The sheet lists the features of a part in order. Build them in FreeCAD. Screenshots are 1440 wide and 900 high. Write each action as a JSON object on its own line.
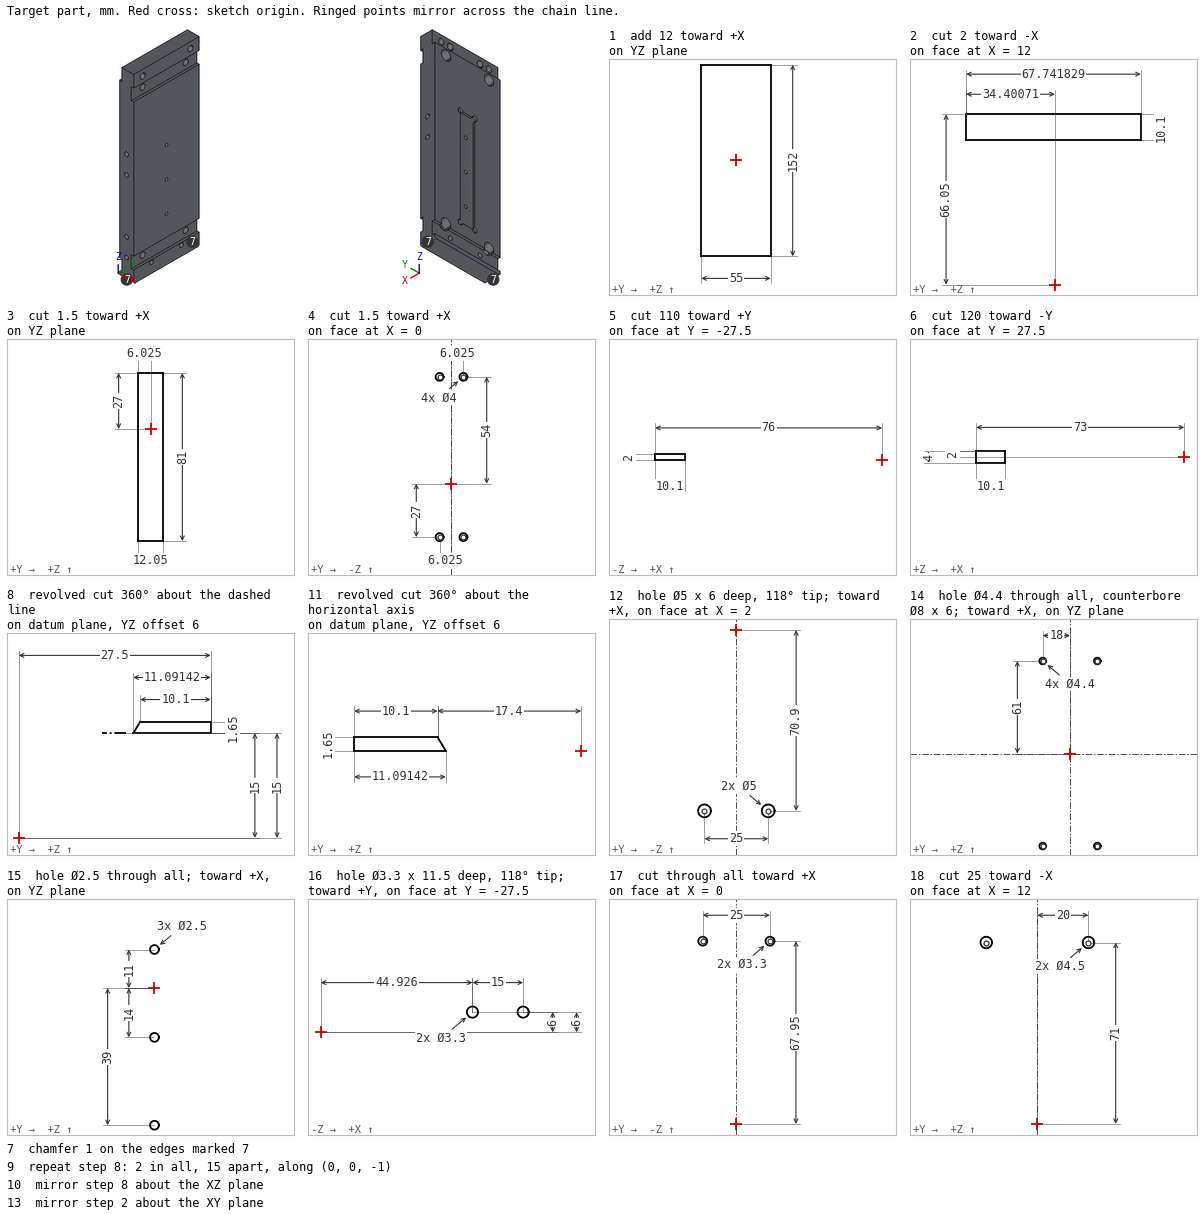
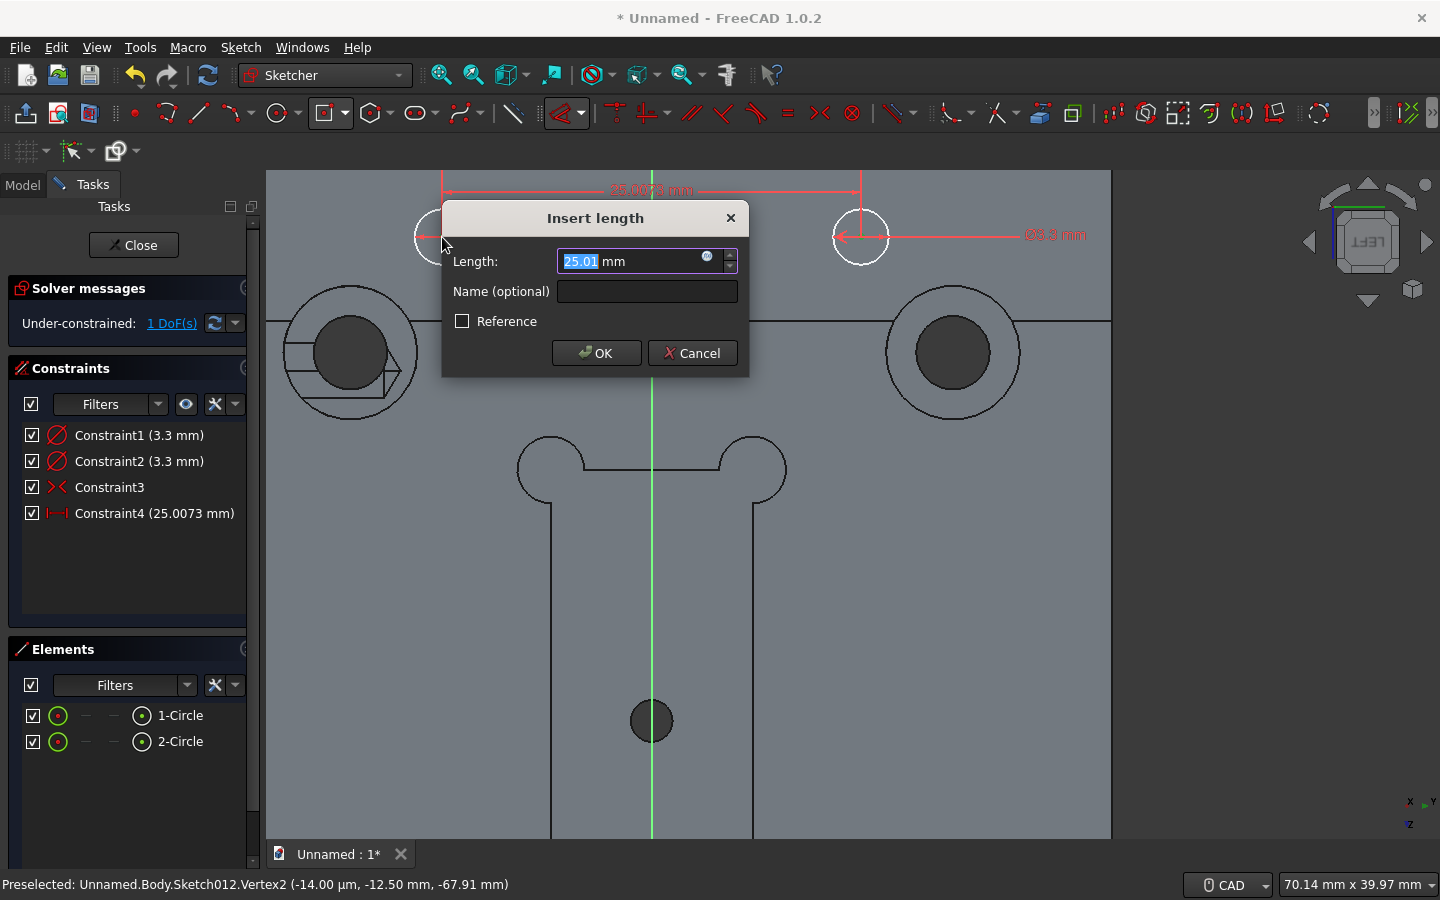
{"action": "type", "text": "25"}
{"action": "key", "text": "Return"}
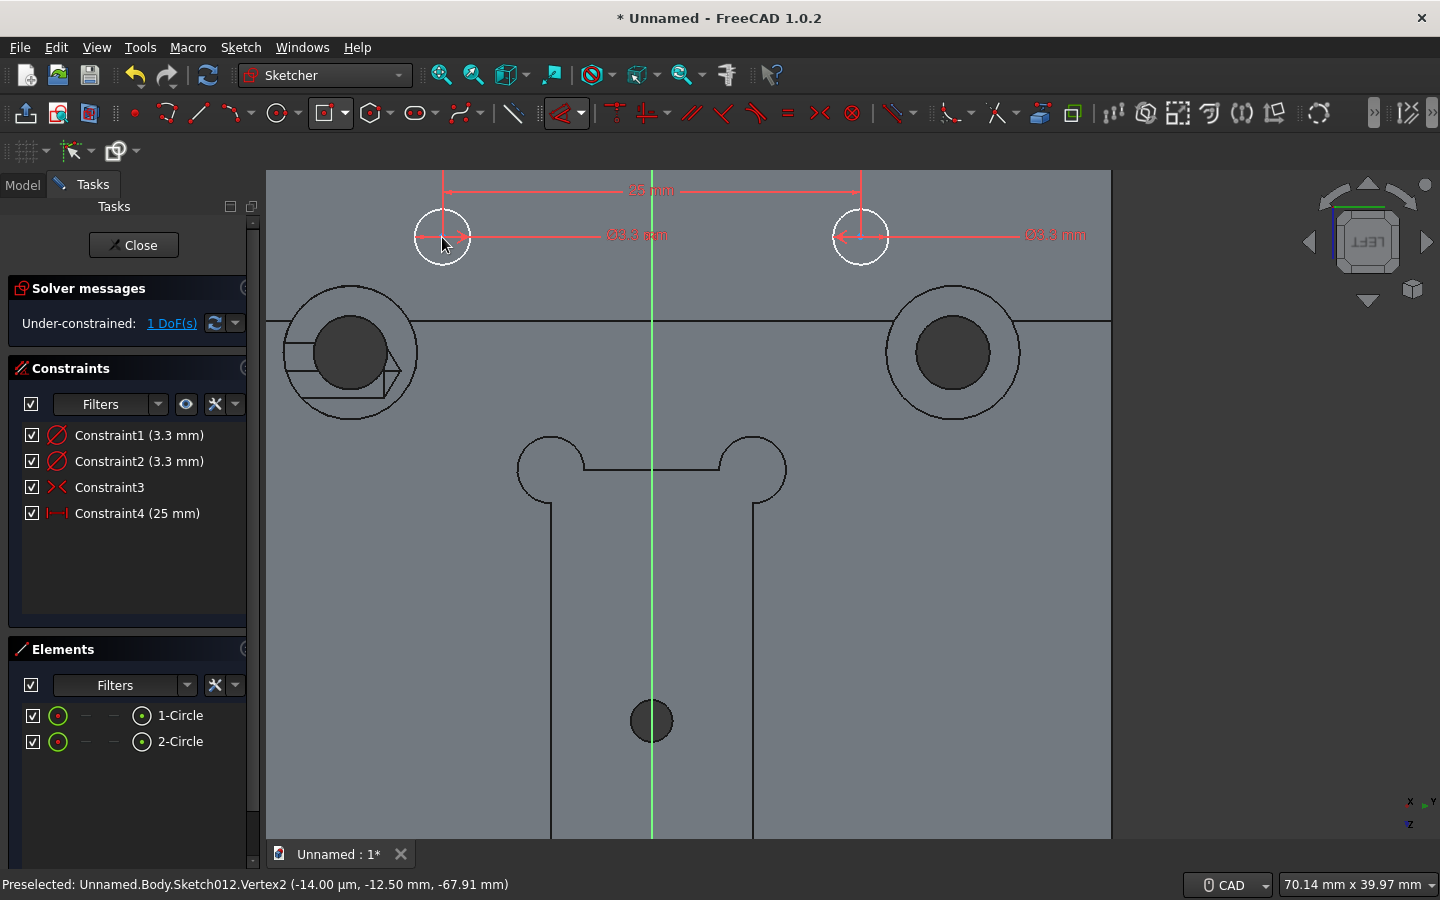
{"action": "left_click", "coordinate": [861, 237]}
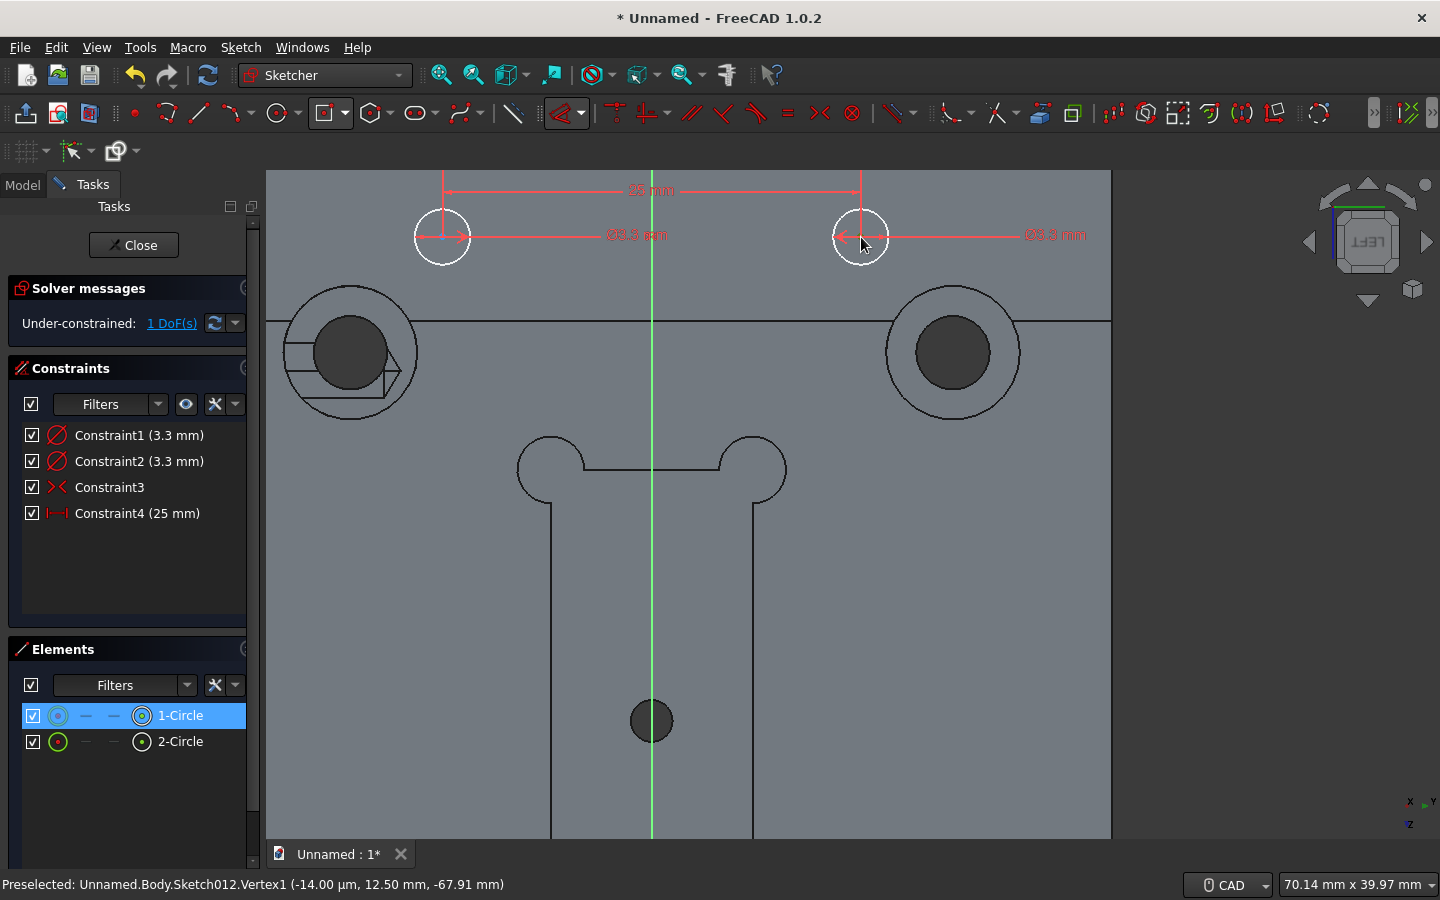
{"action": "left_click", "coordinate": [584, 114]}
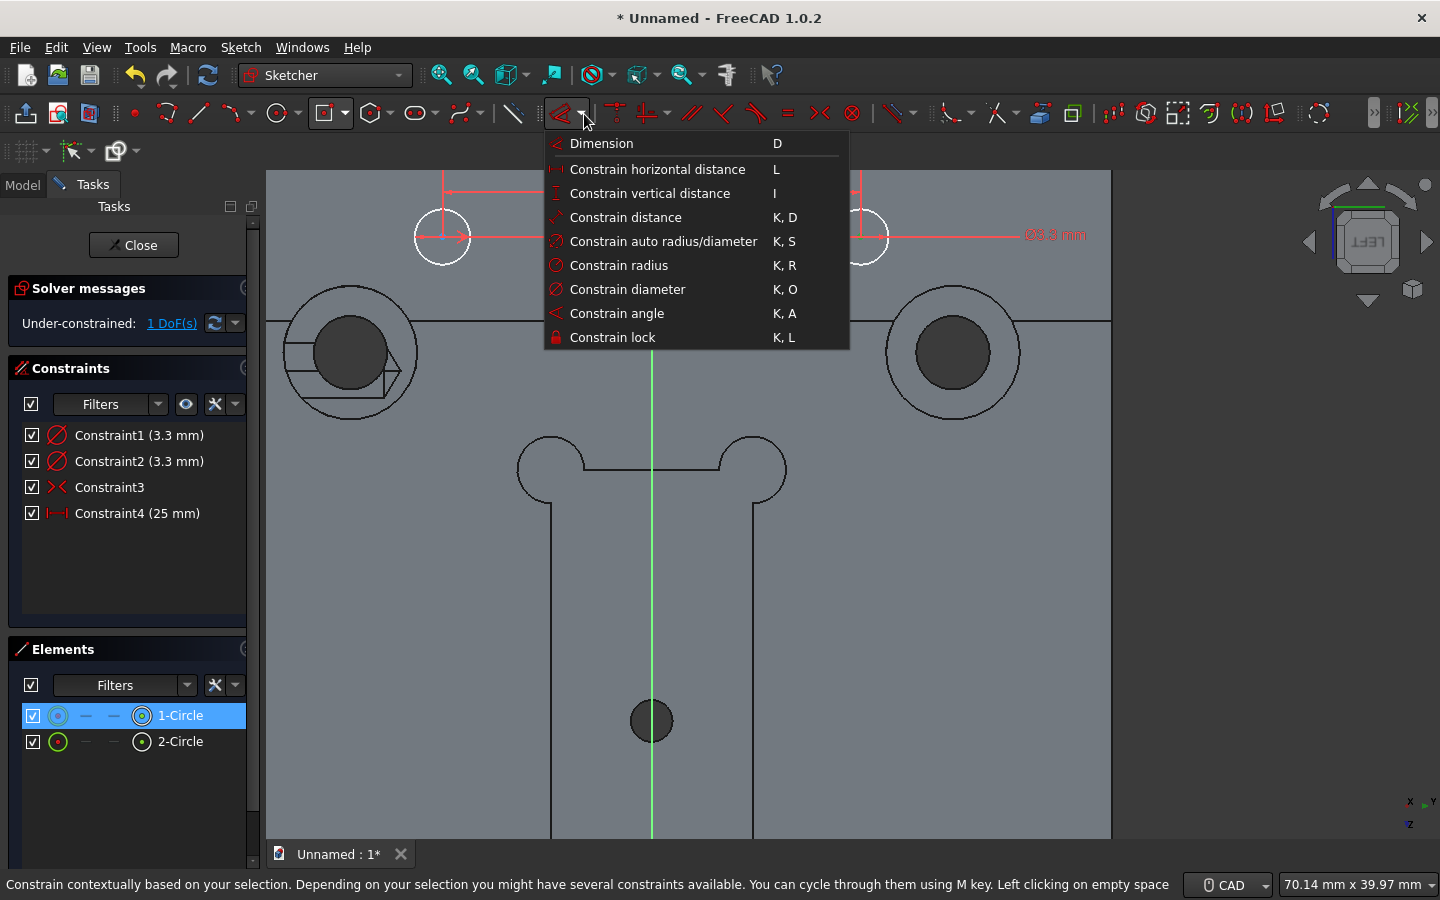
{"action": "left_click", "coordinate": [697, 193]}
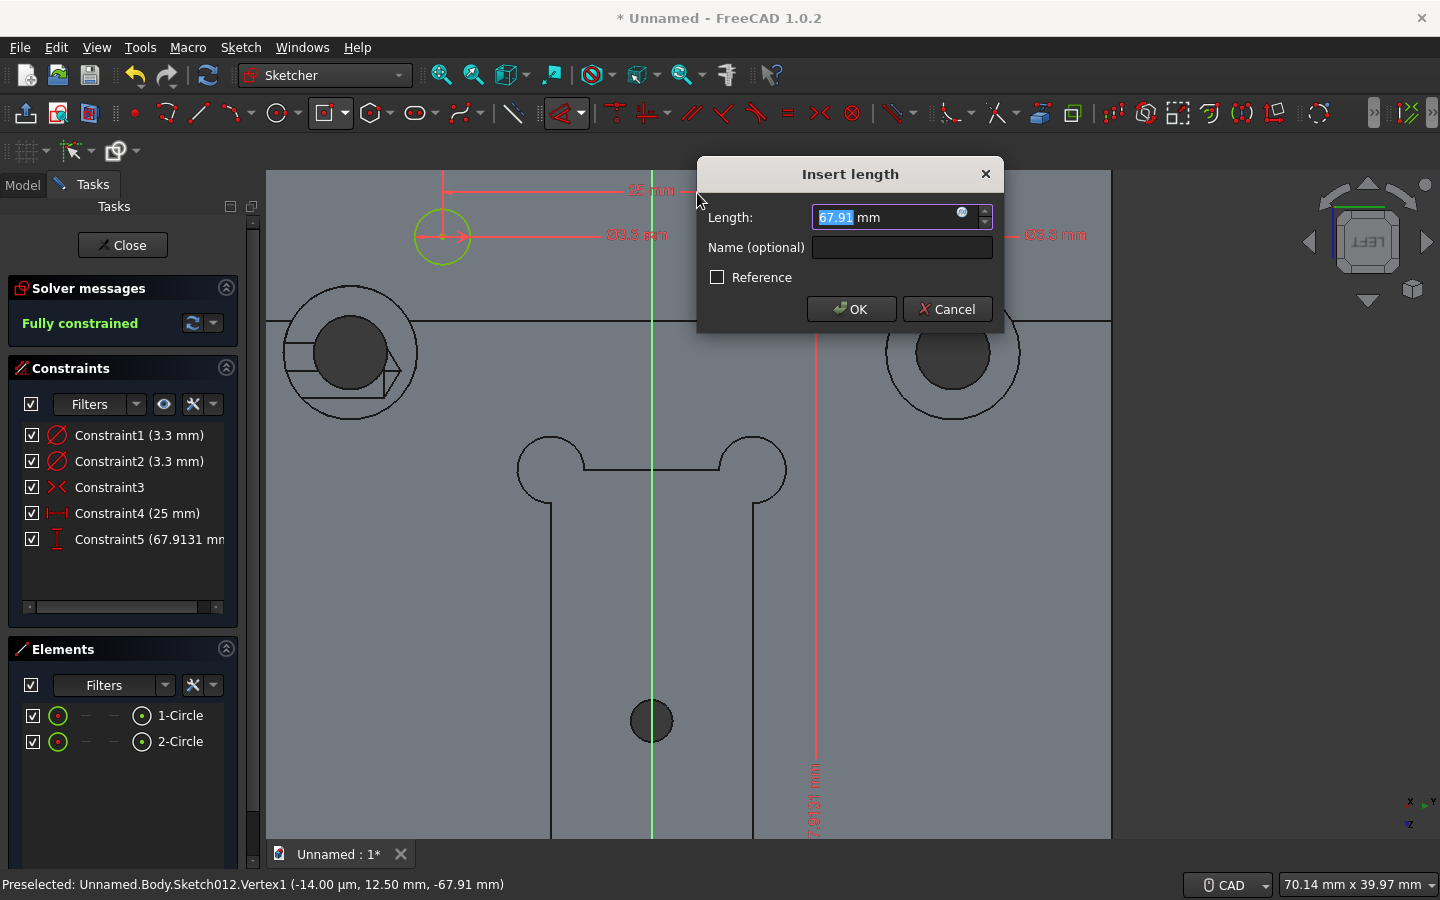
{"action": "type", "text": "67.95"}
{"action": "key", "text": "Return"}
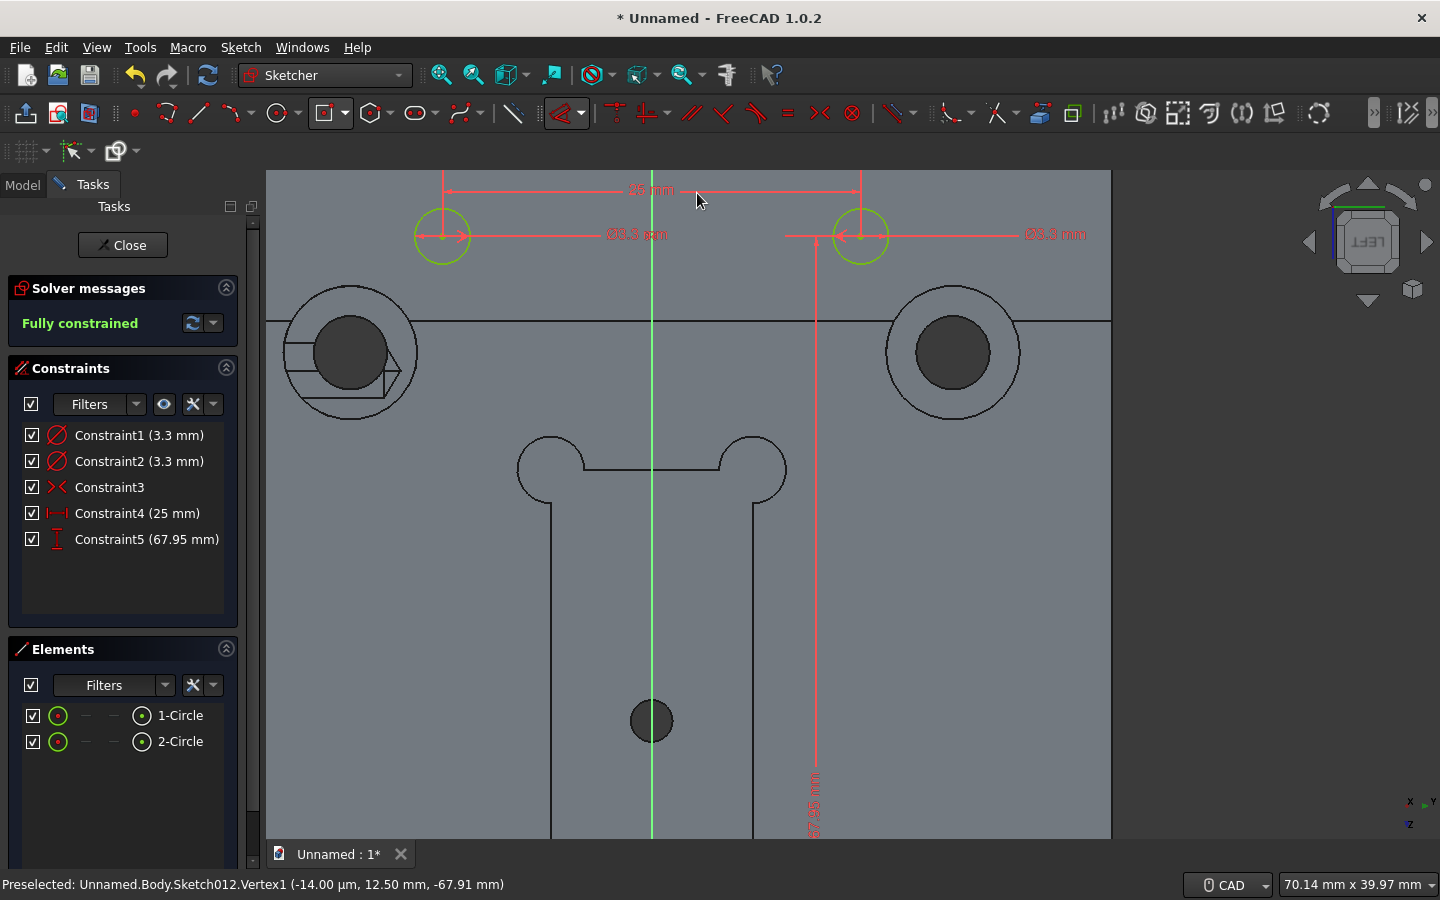
{"action": "left_click", "coordinate": [123, 245]}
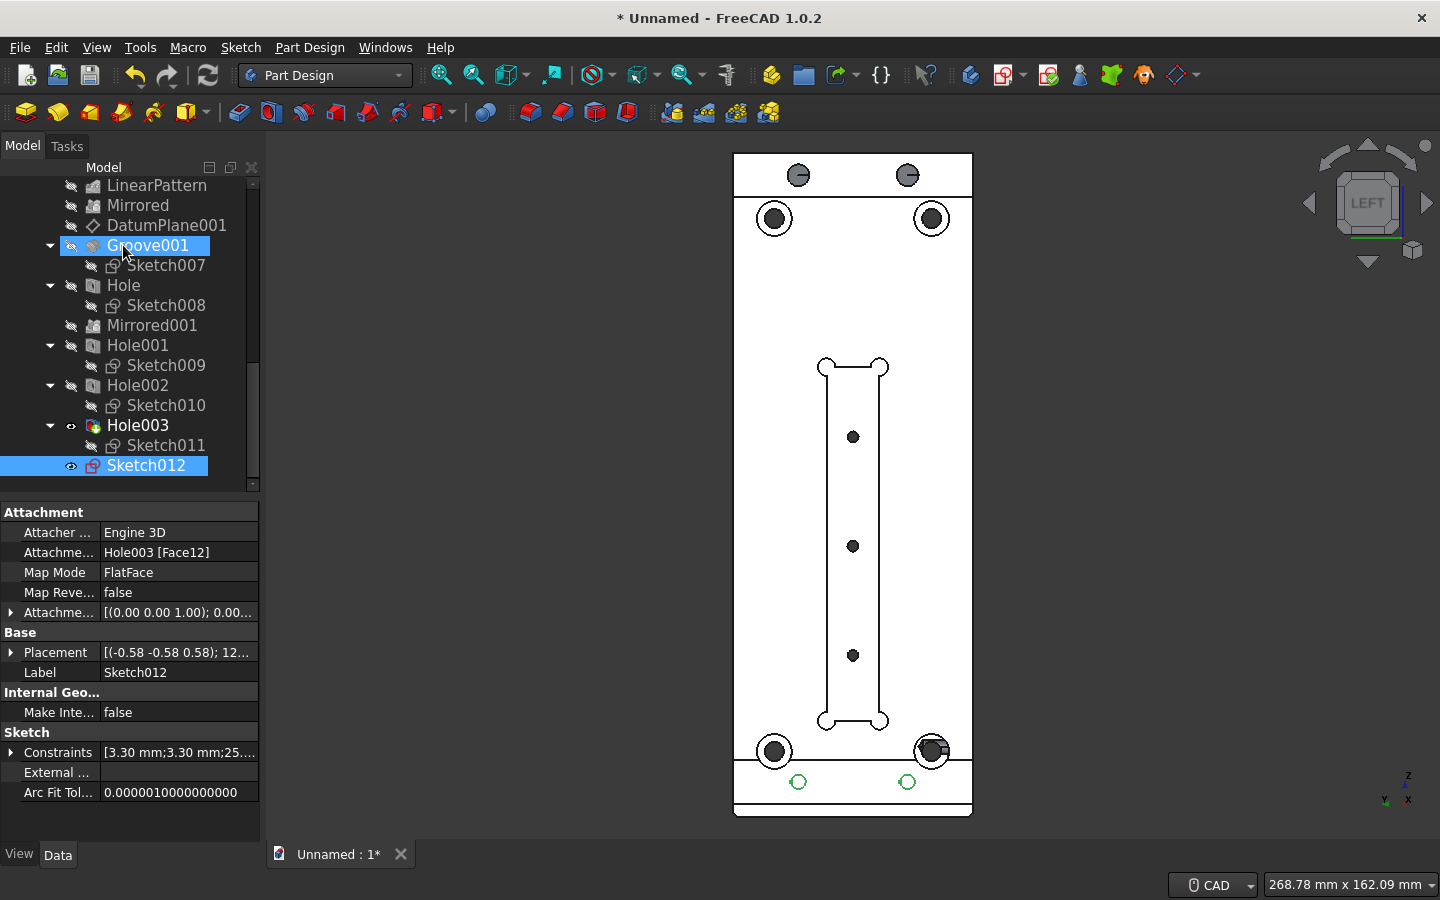
{"action": "left_click", "coordinate": [240, 112]}